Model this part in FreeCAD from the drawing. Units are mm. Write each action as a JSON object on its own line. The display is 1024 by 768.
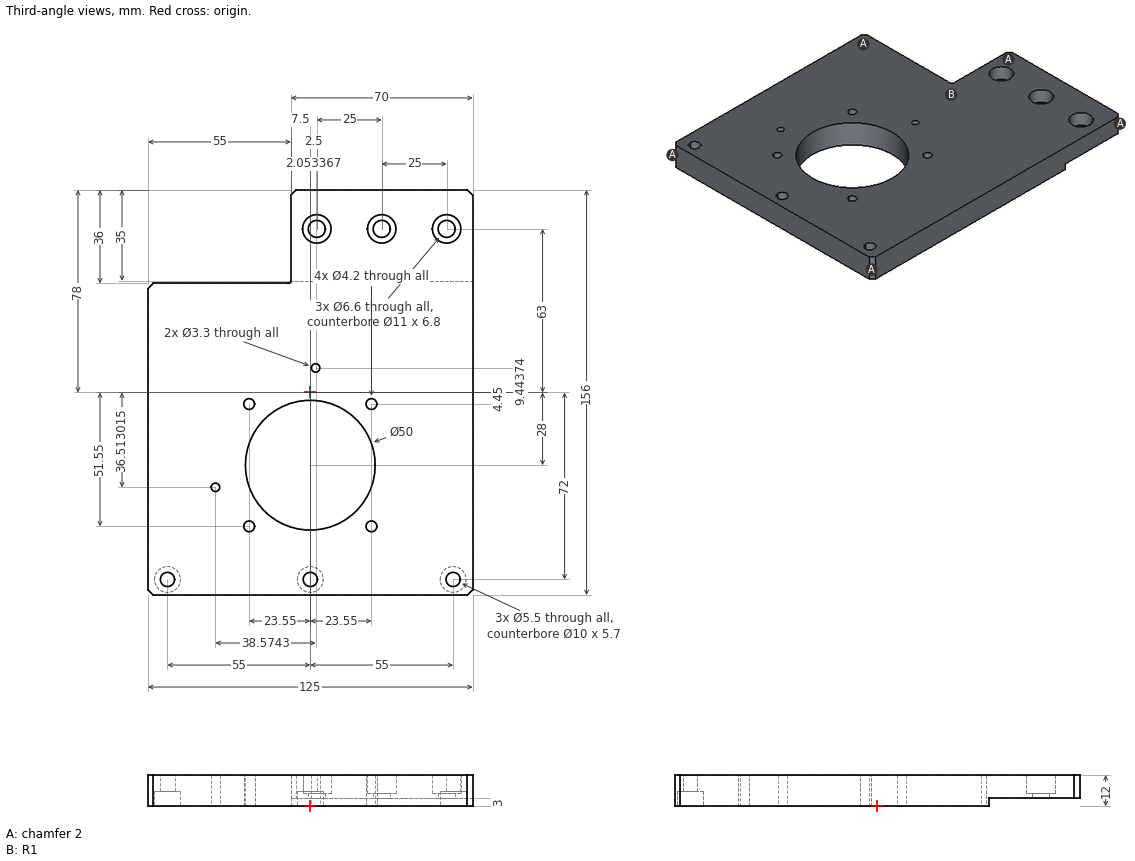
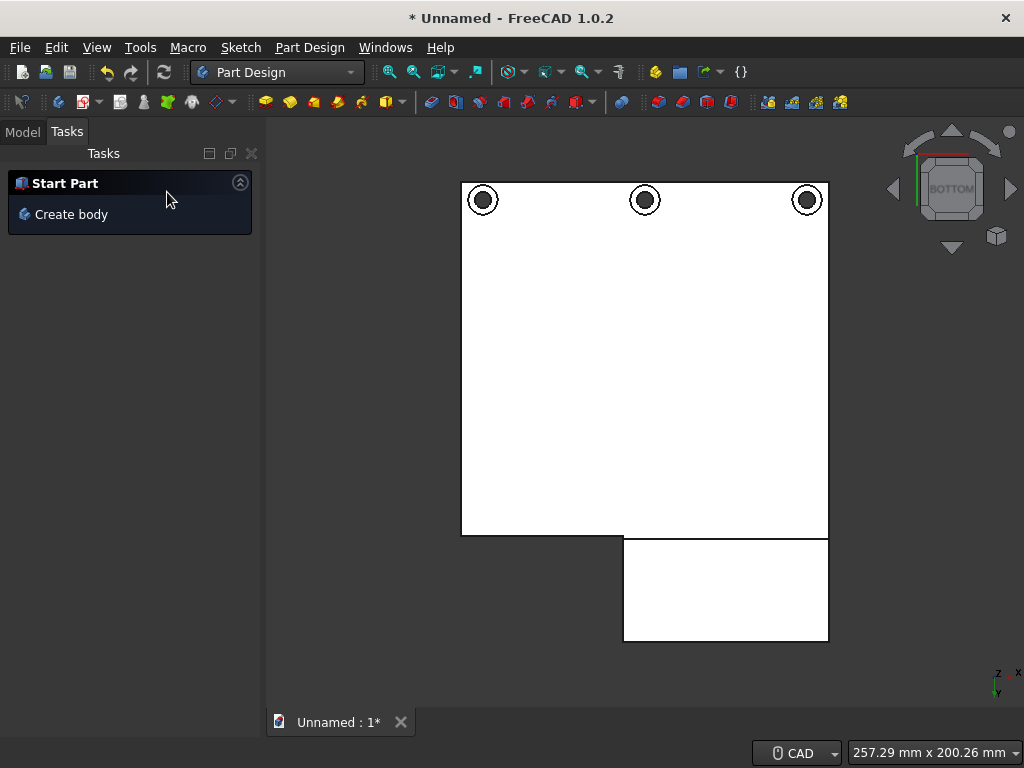
{"action": "key", "text": "0"}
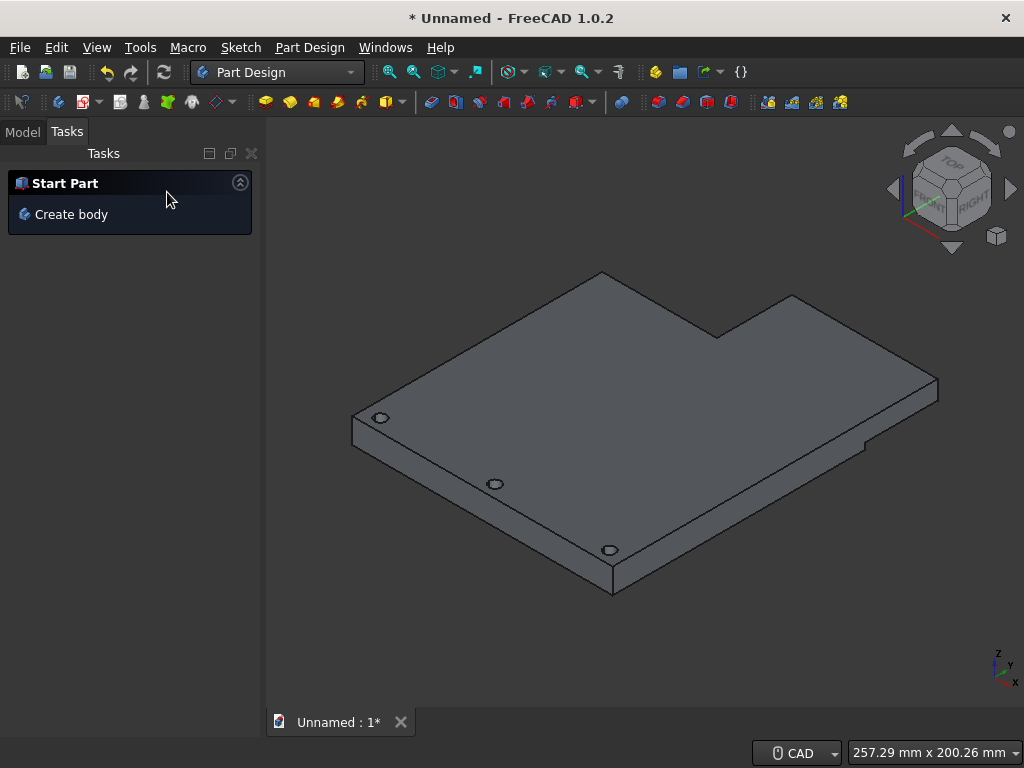
{"action": "left_click", "coordinate": [599, 423]}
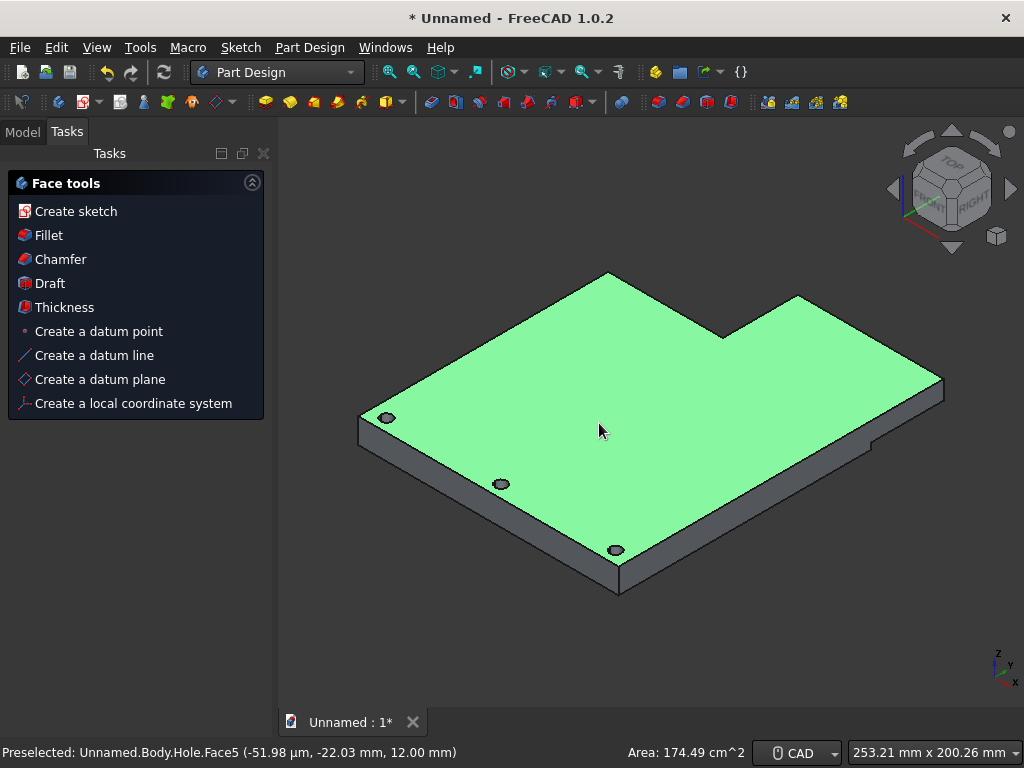
{"action": "left_click", "coordinate": [84, 102]}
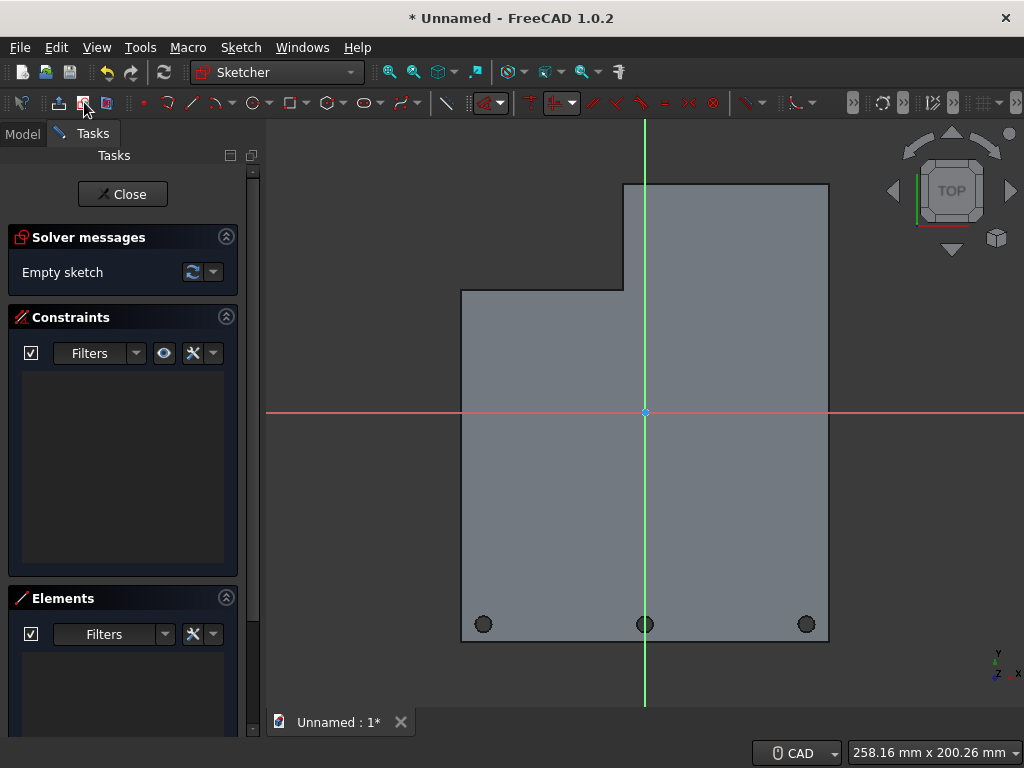
{"action": "scroll", "coordinate": [859, 197], "scroll_direction": "up", "scroll_amount": 3}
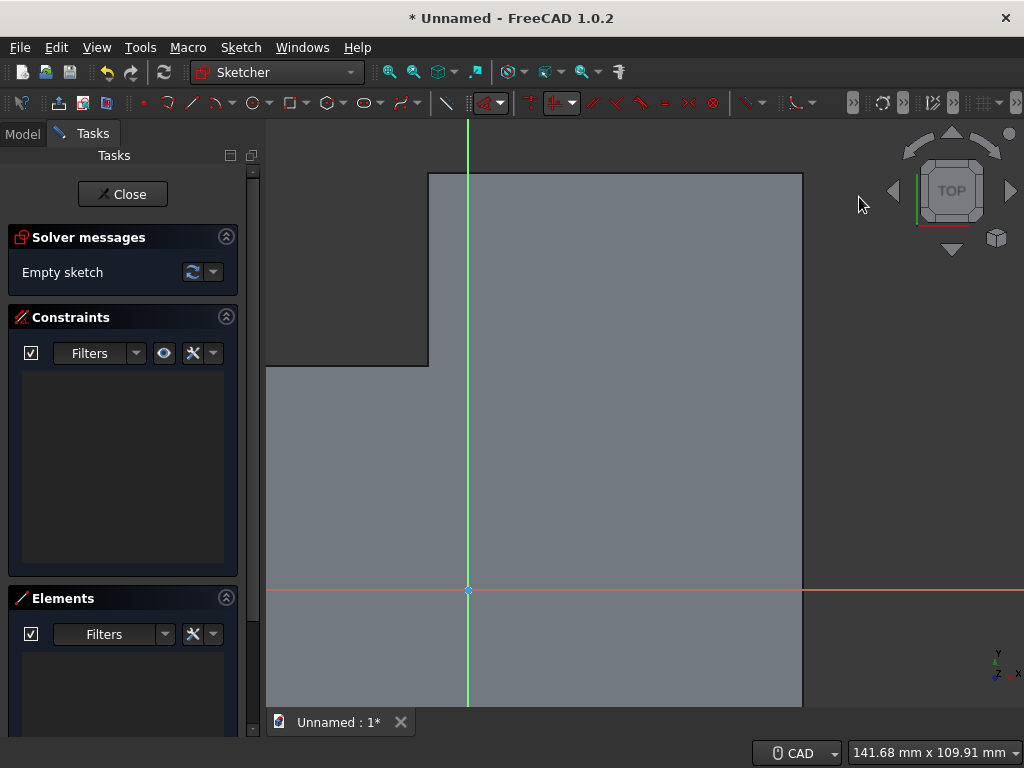
{"action": "left_click", "coordinate": [254, 104]}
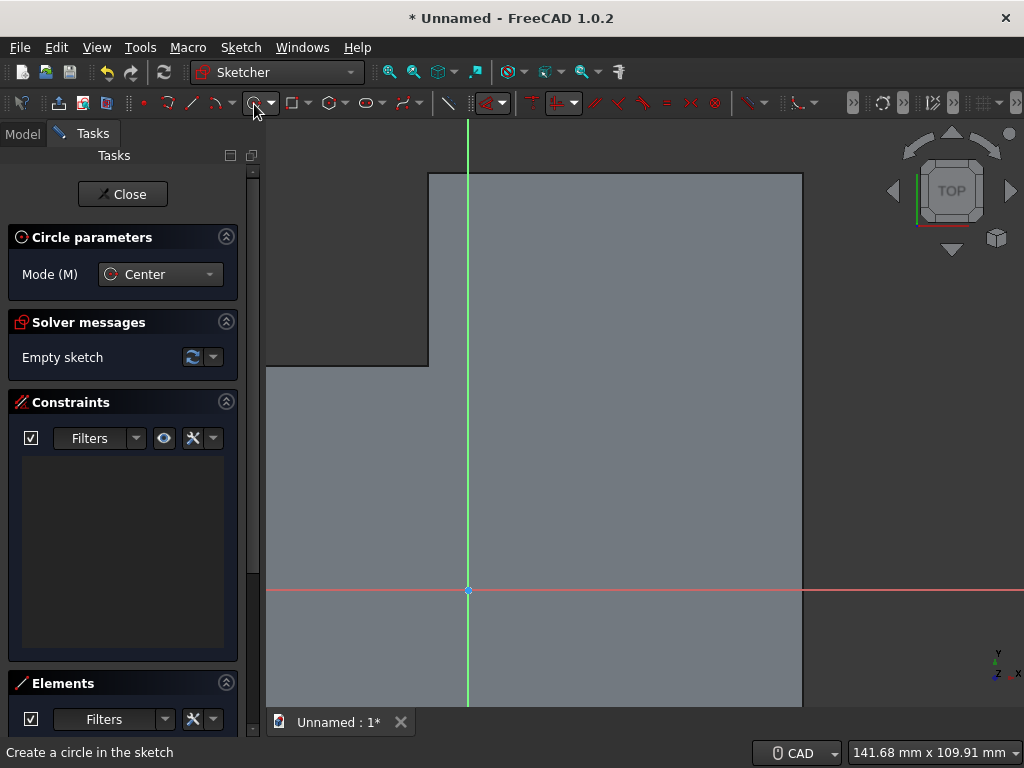
{"action": "scroll", "coordinate": [749, 253], "scroll_direction": "up", "scroll_amount": 2}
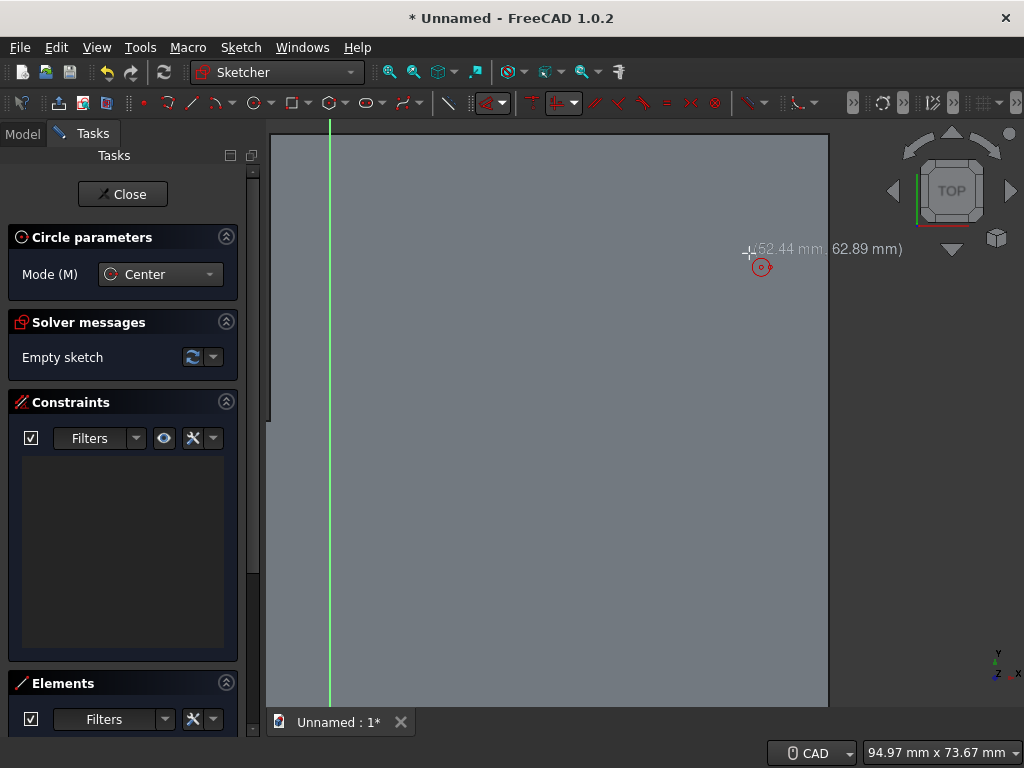
{"action": "left_click", "coordinate": [749, 254]}
{"action": "left_click", "coordinate": [768, 235]}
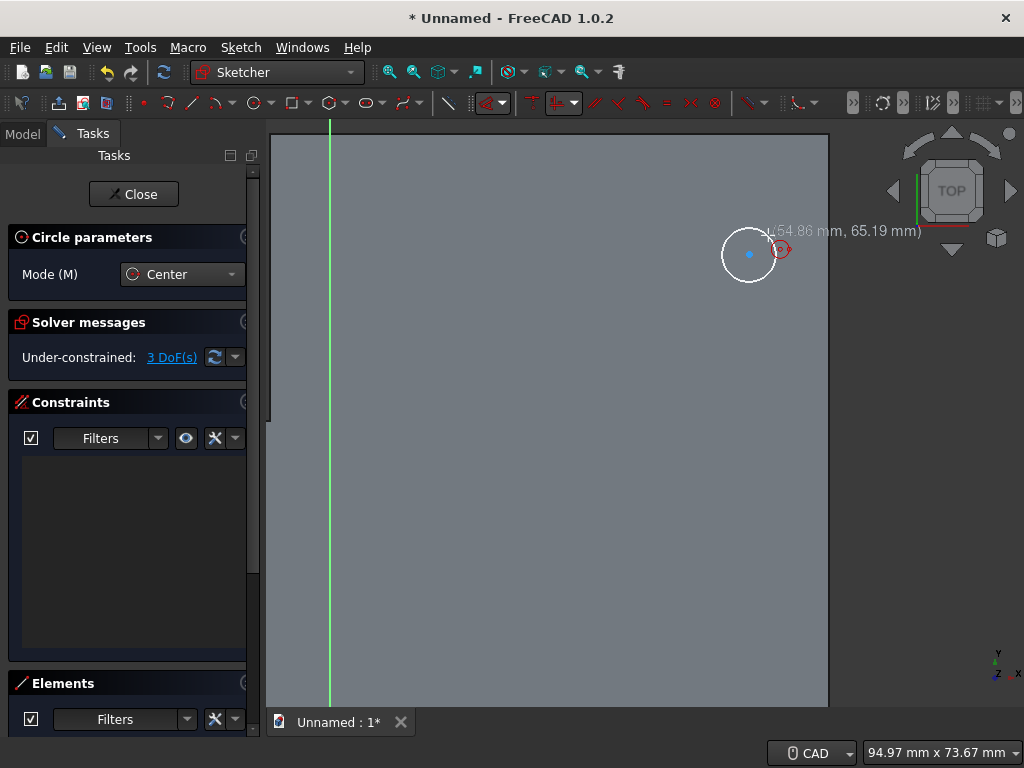
{"action": "left_click", "coordinate": [550, 254]}
{"action": "left_click", "coordinate": [568, 235]}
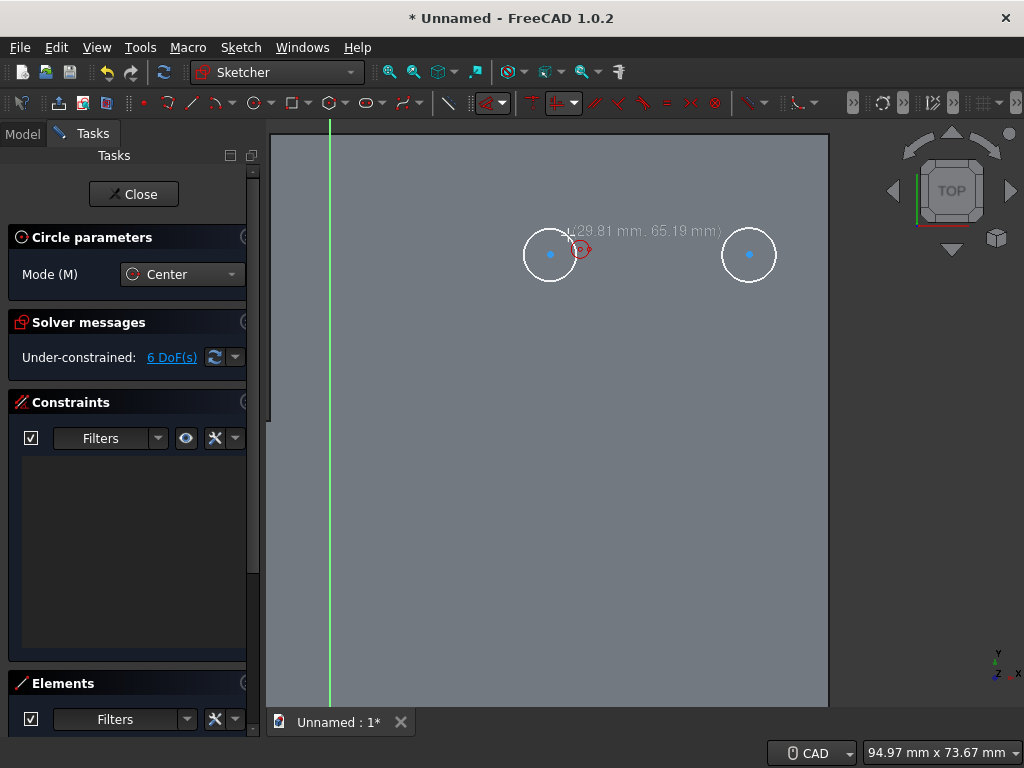
{"action": "left_click", "coordinate": [350, 254]}
{"action": "left_click", "coordinate": [369, 235]}
{"action": "key", "text": "Escape"}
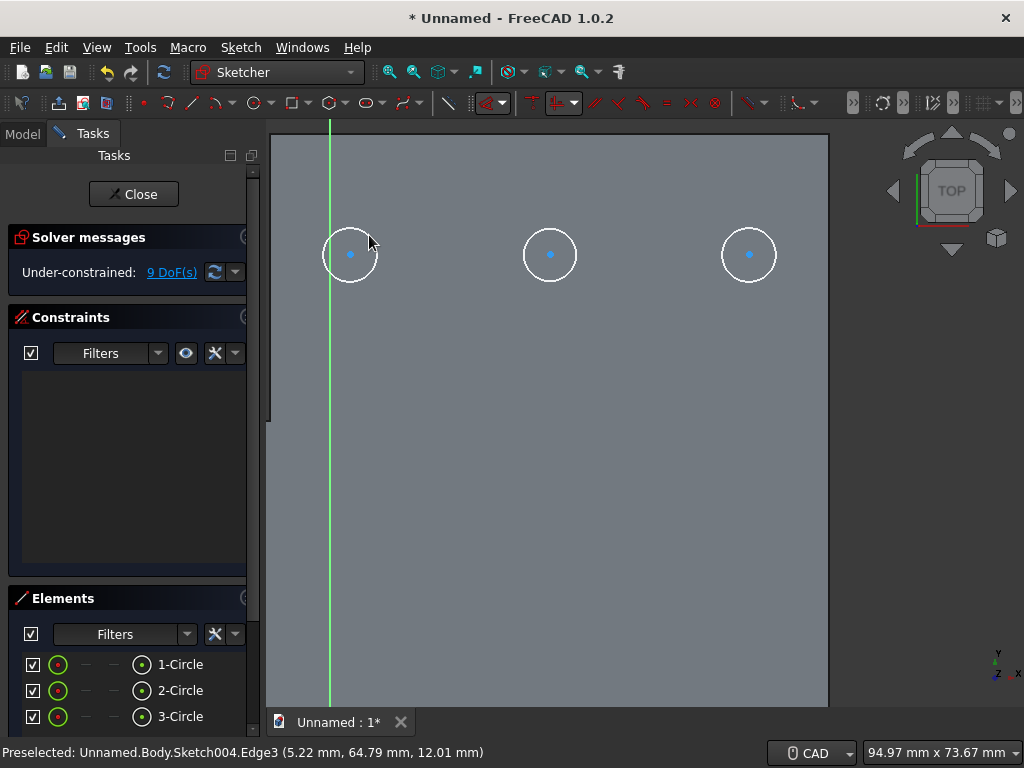
{"action": "left_click", "coordinate": [768, 236]}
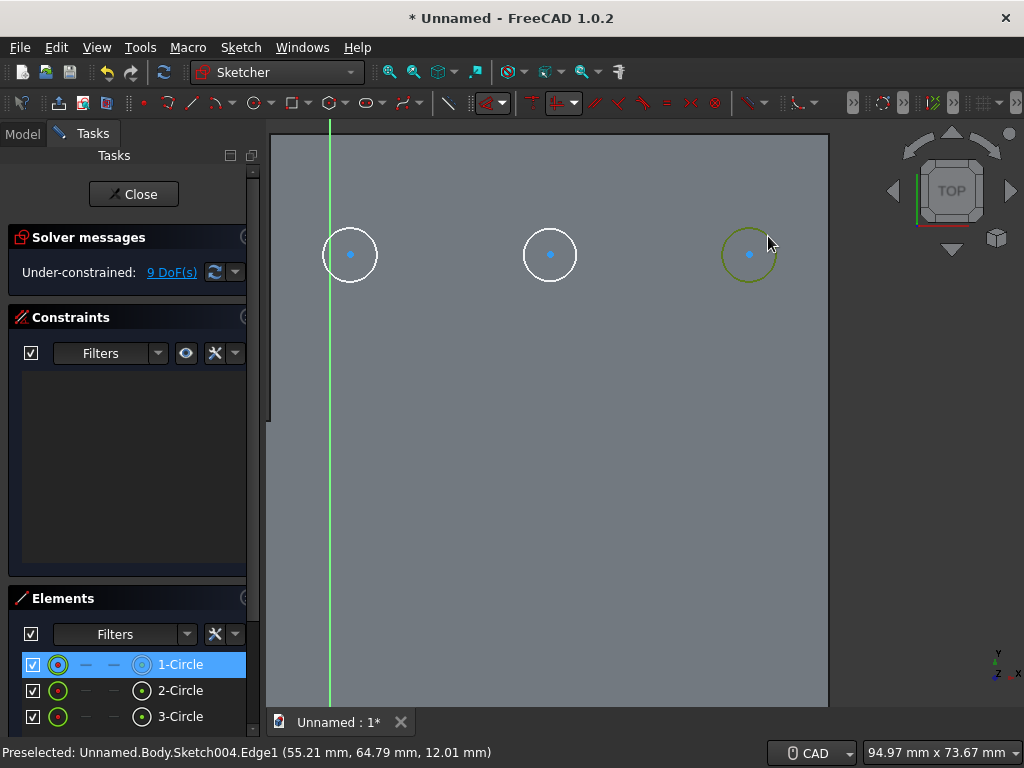
{"action": "left_click", "coordinate": [568, 236]}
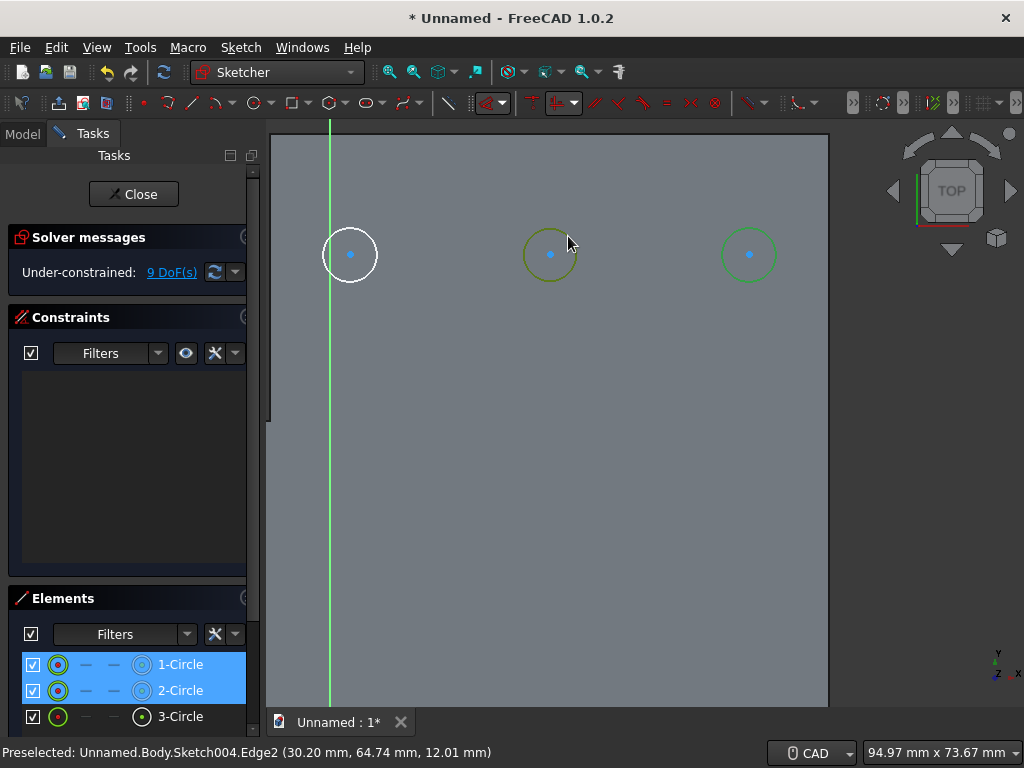
{"action": "left_click", "coordinate": [369, 236]}